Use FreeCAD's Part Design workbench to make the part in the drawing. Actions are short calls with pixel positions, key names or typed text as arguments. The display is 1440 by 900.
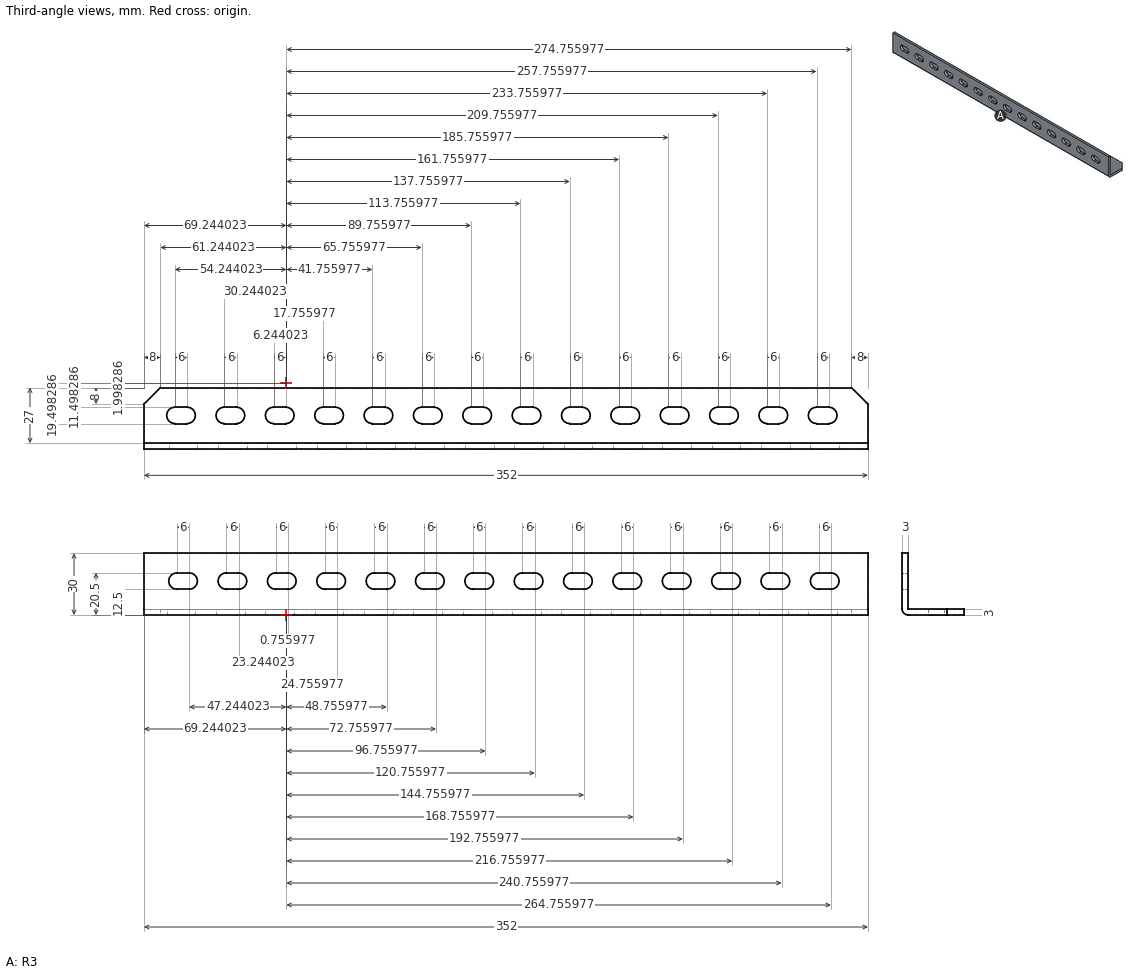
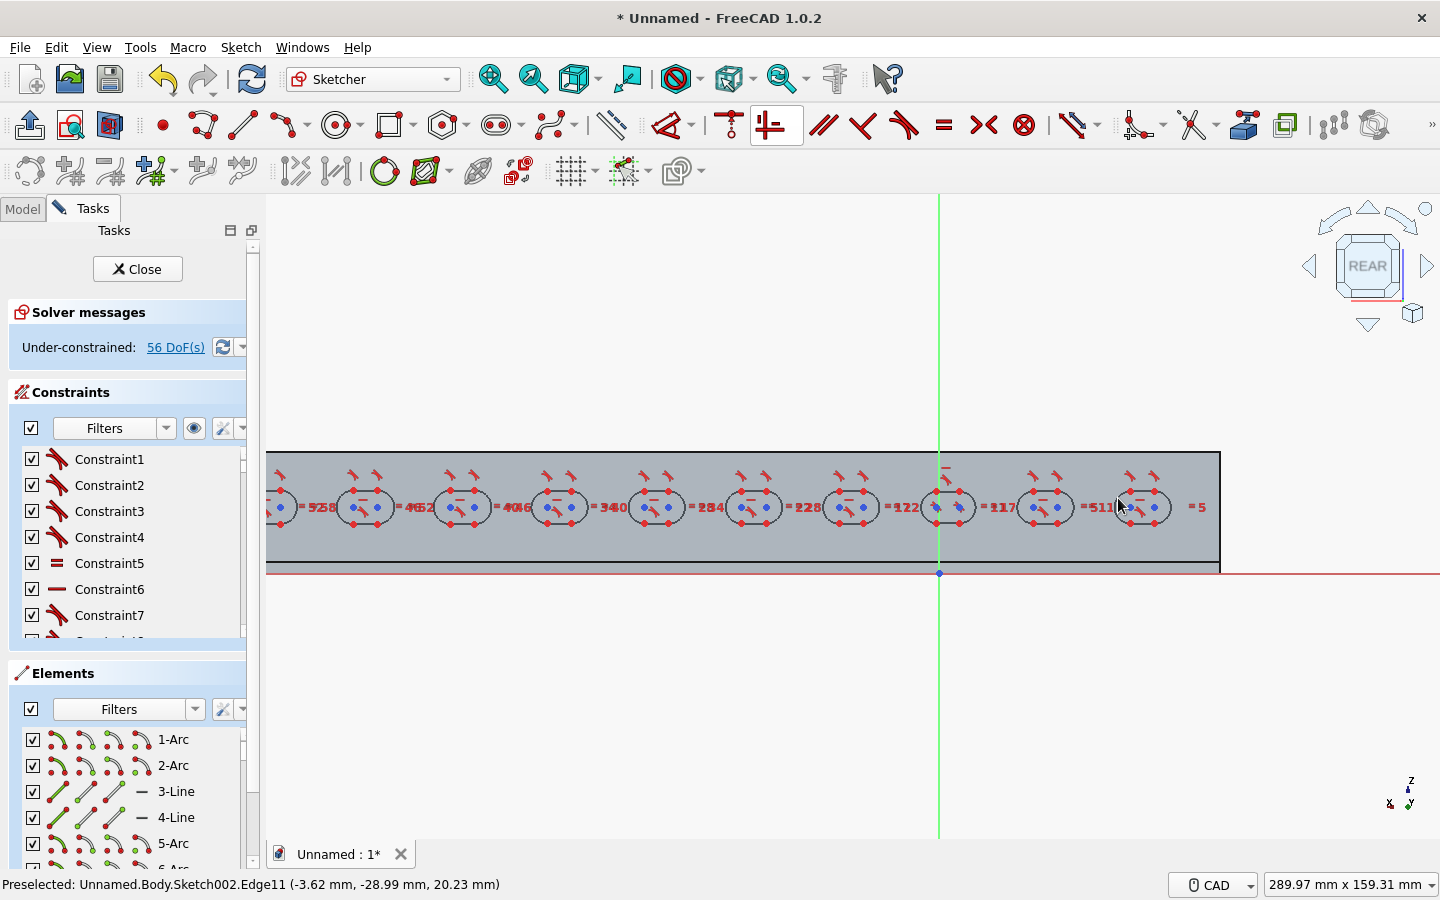
click(1118, 498)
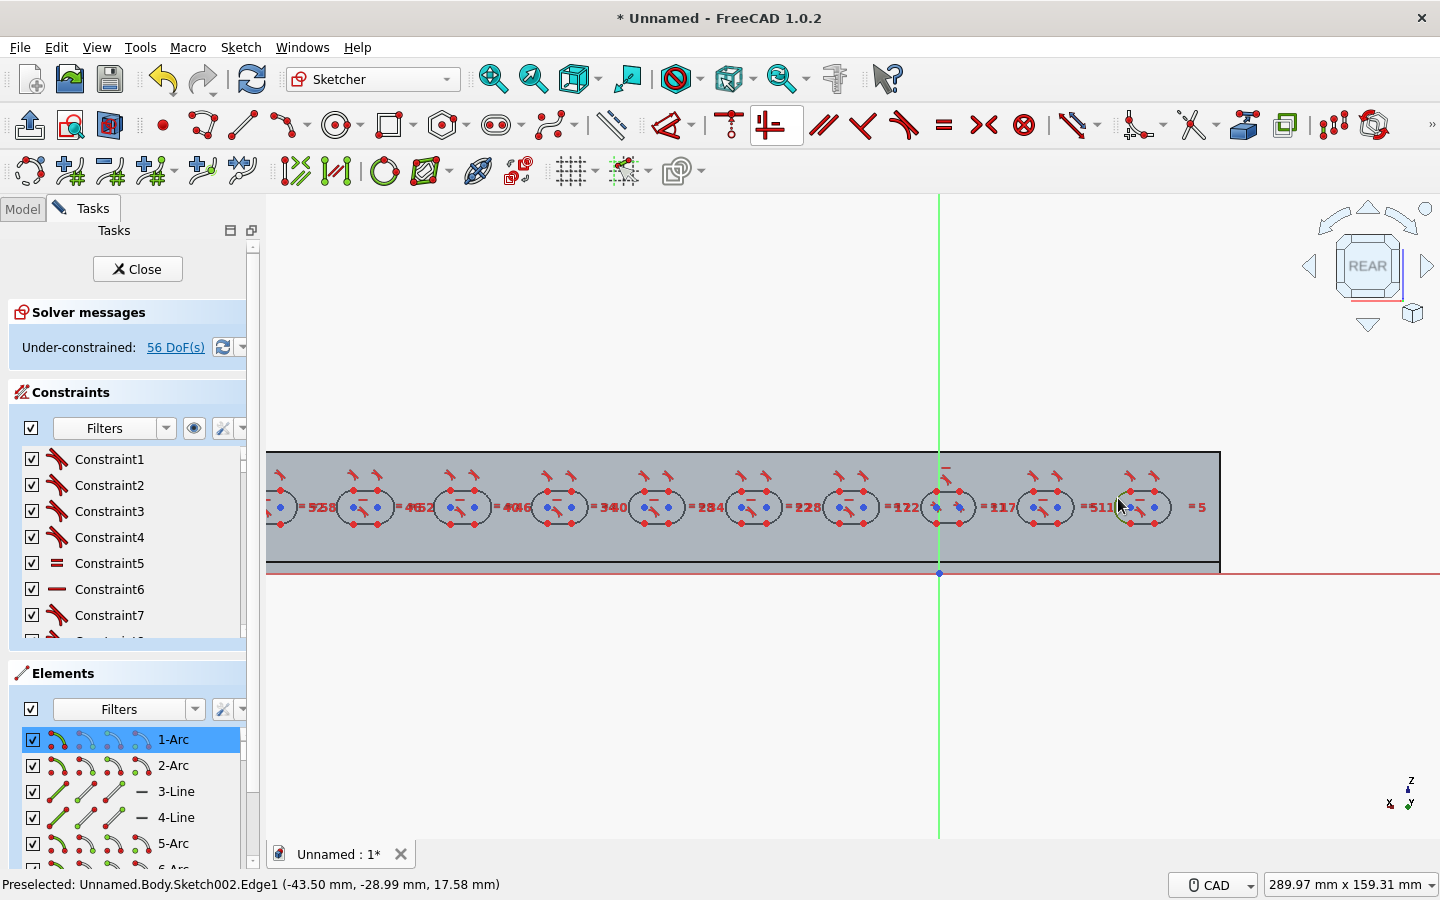
click(1020, 498)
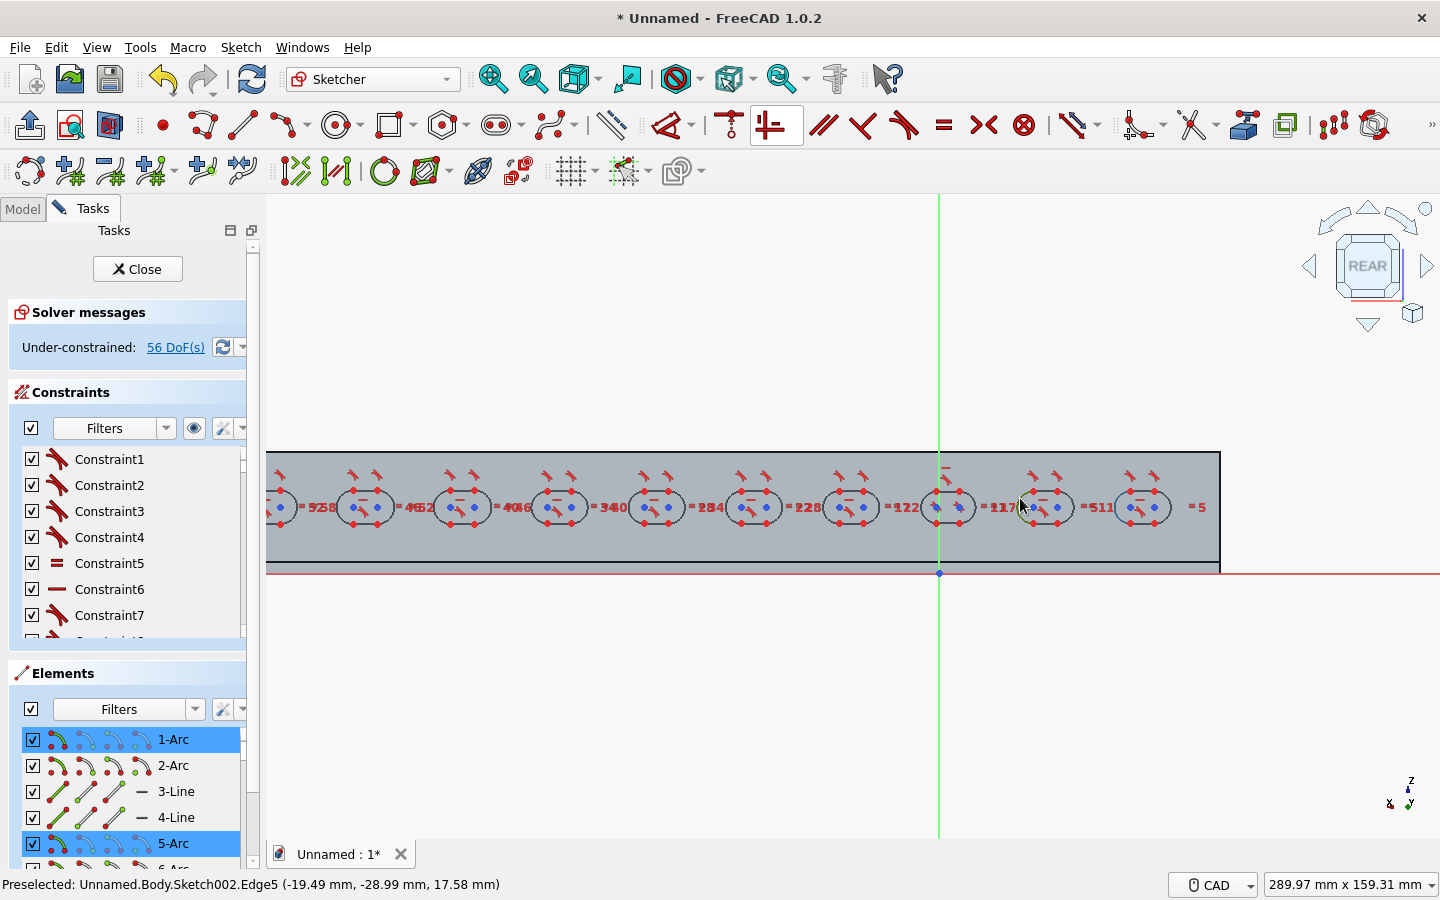
click(924, 498)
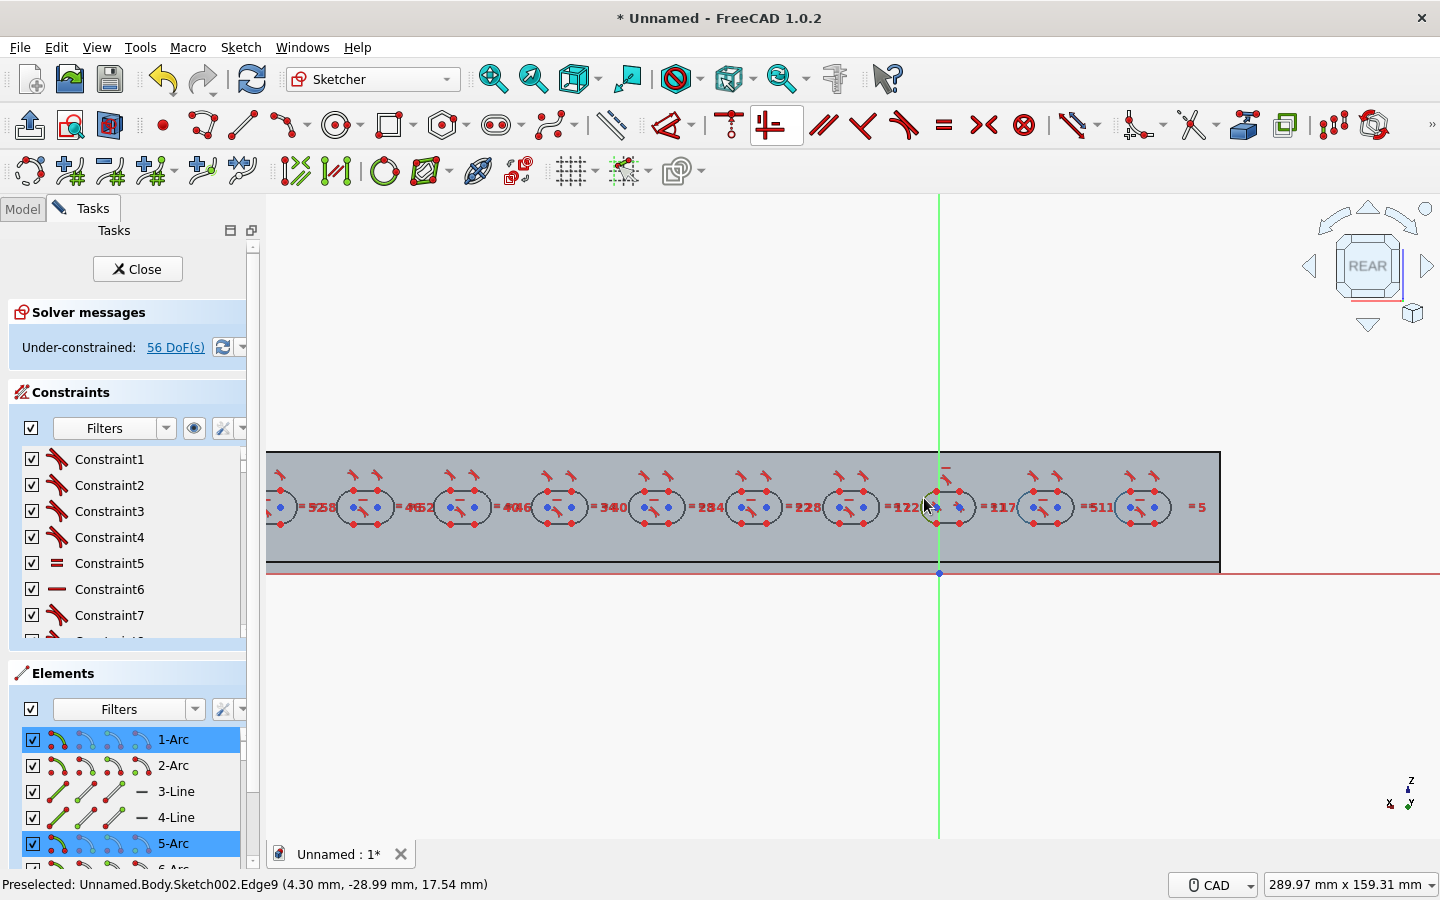
click(826, 498)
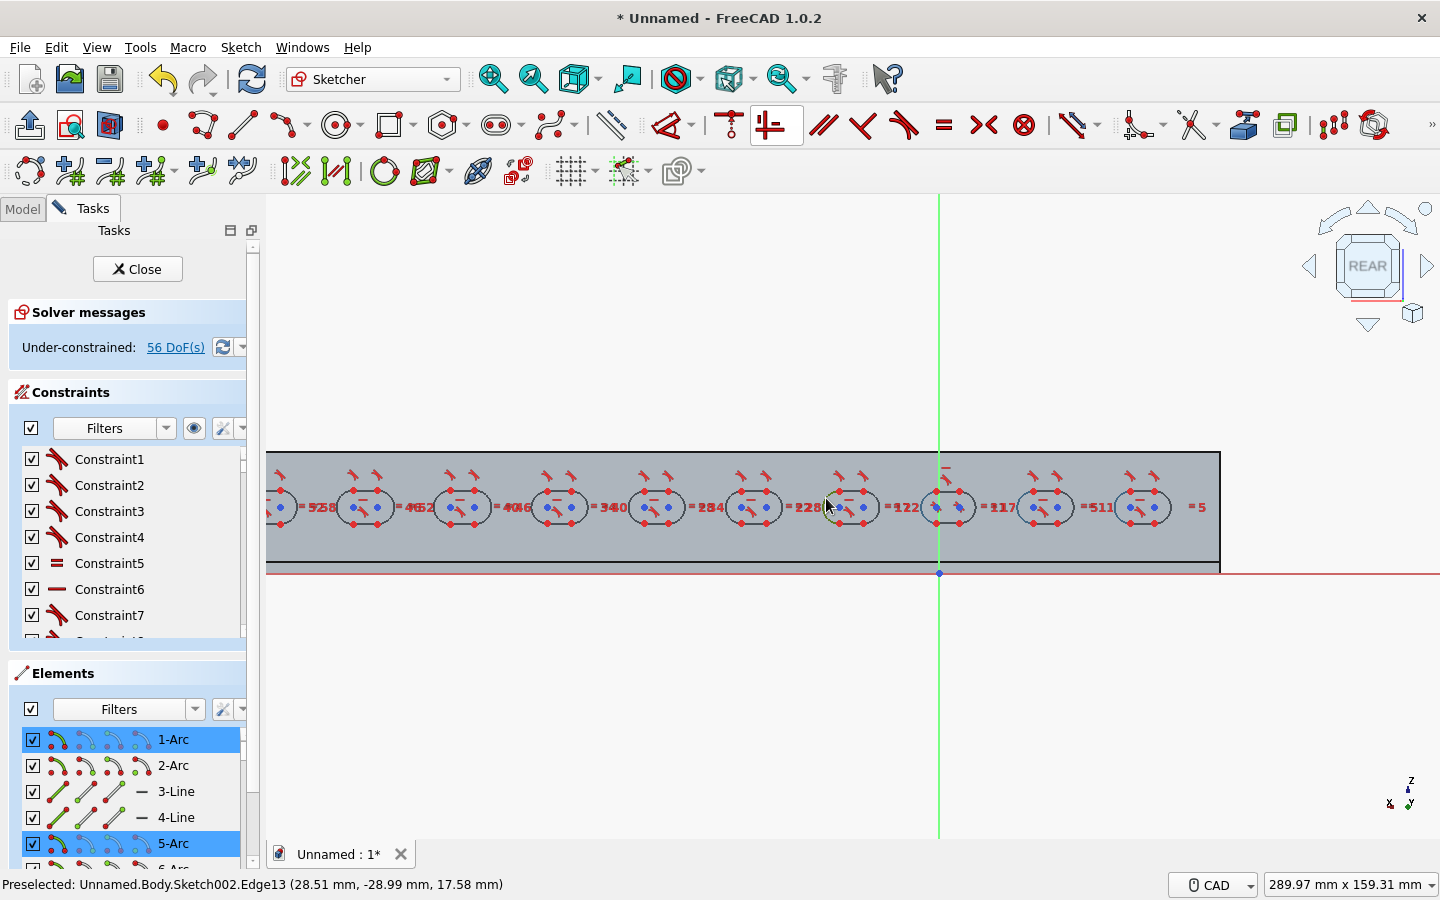
click(729, 498)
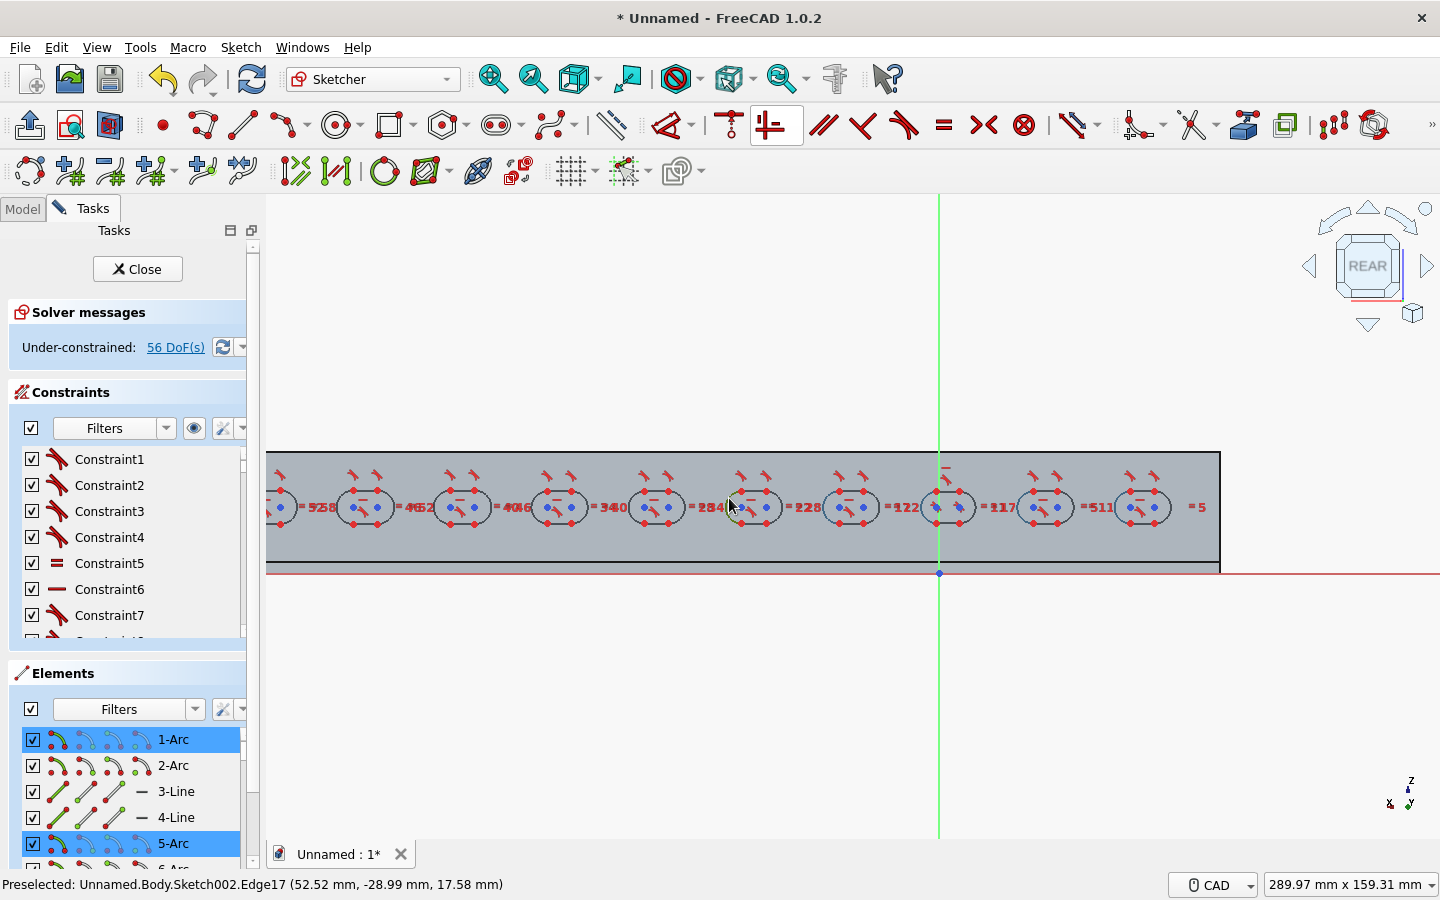
click(632, 498)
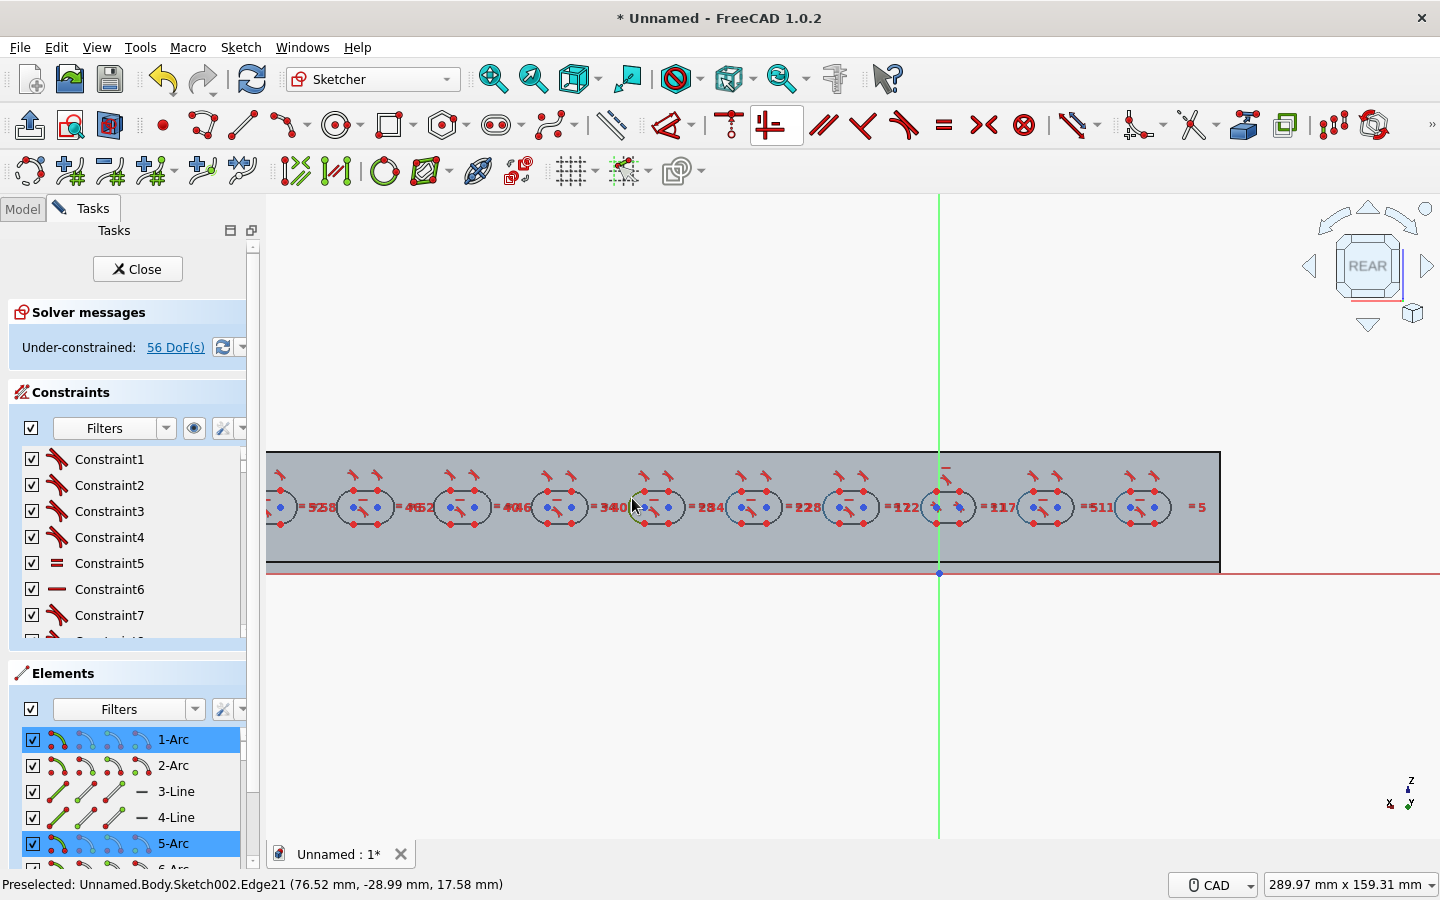
click(534, 498)